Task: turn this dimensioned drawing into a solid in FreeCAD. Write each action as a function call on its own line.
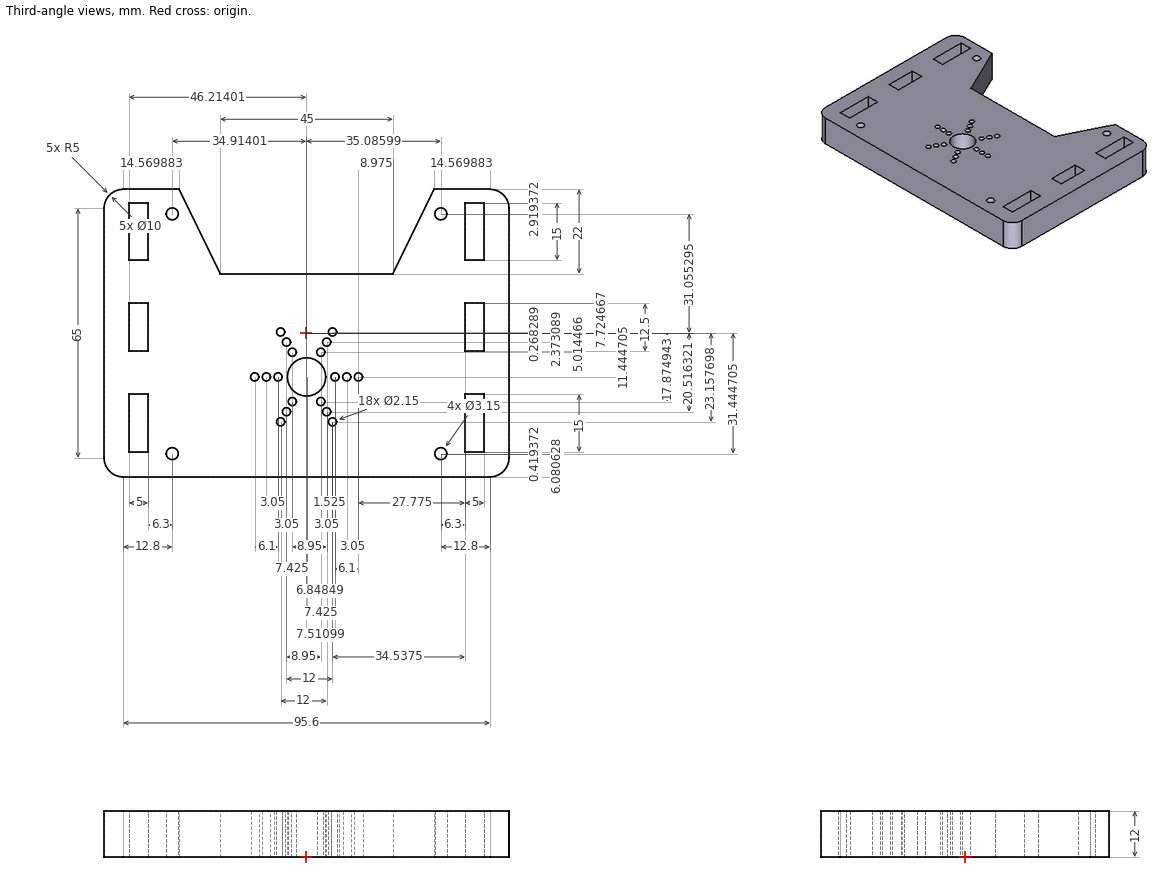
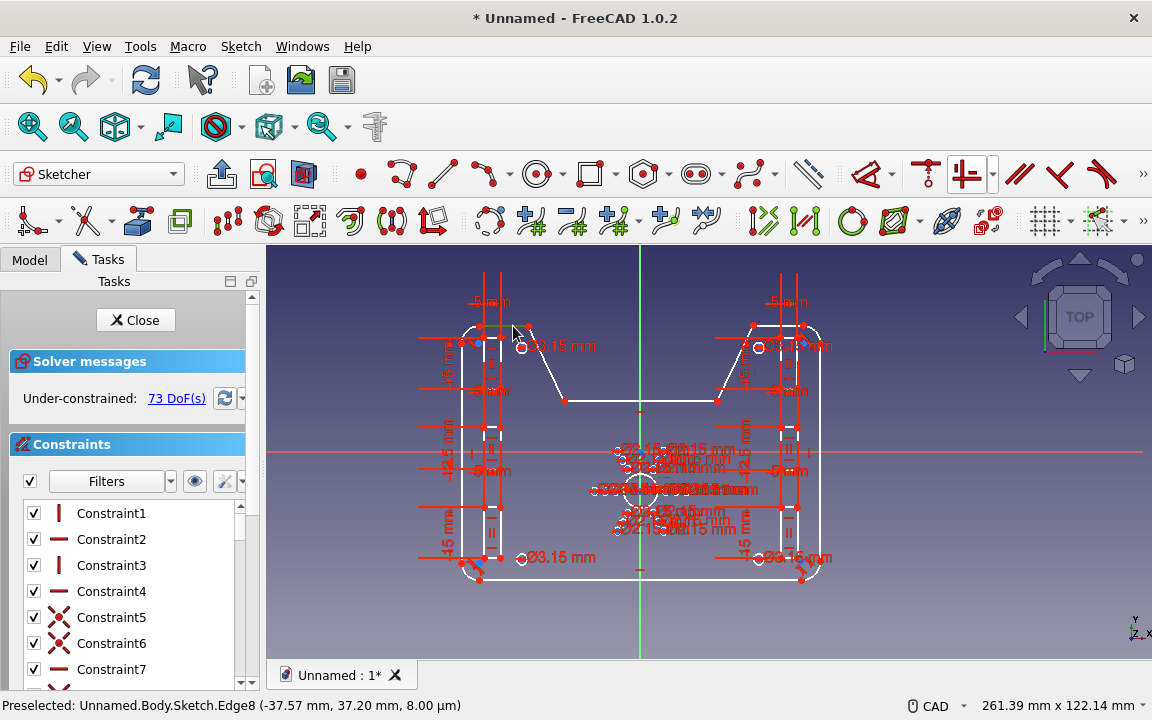
click(467, 331)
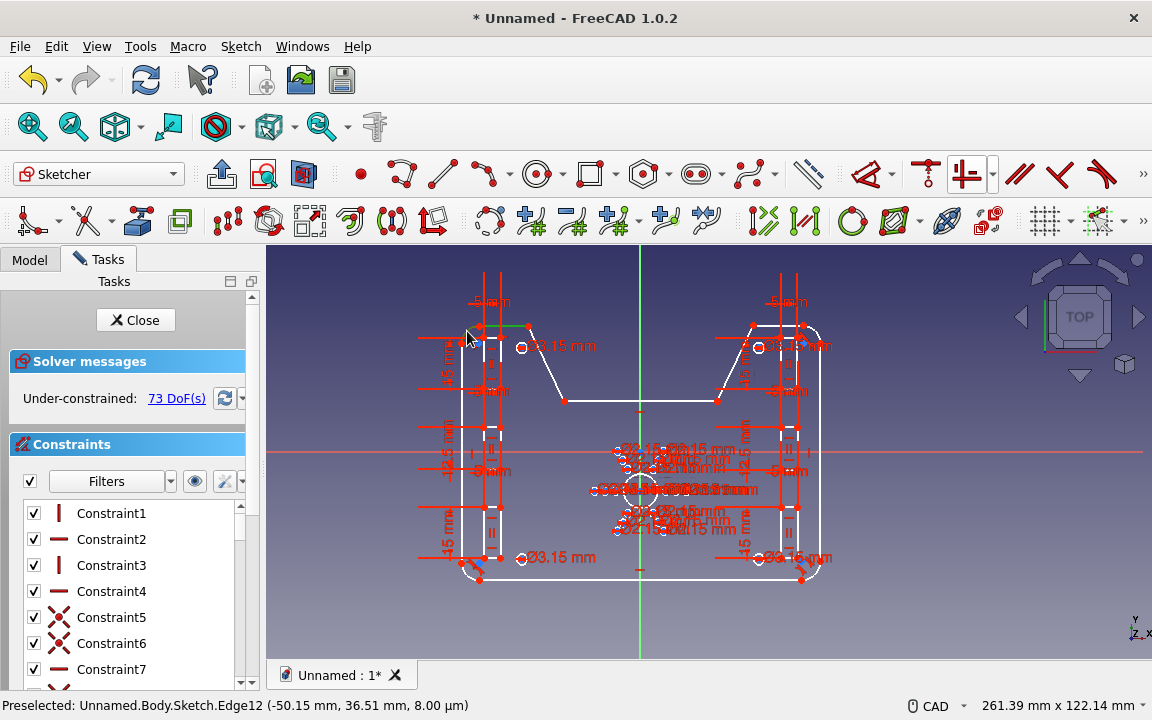
click(1102, 174)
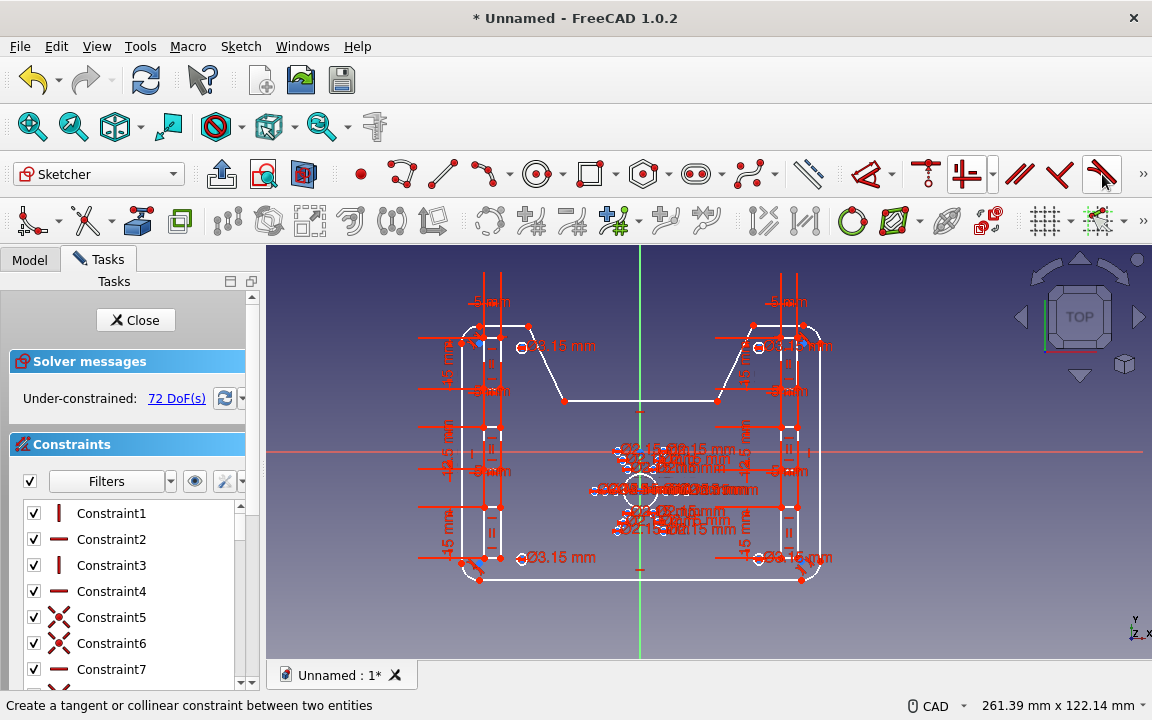
click(467, 575)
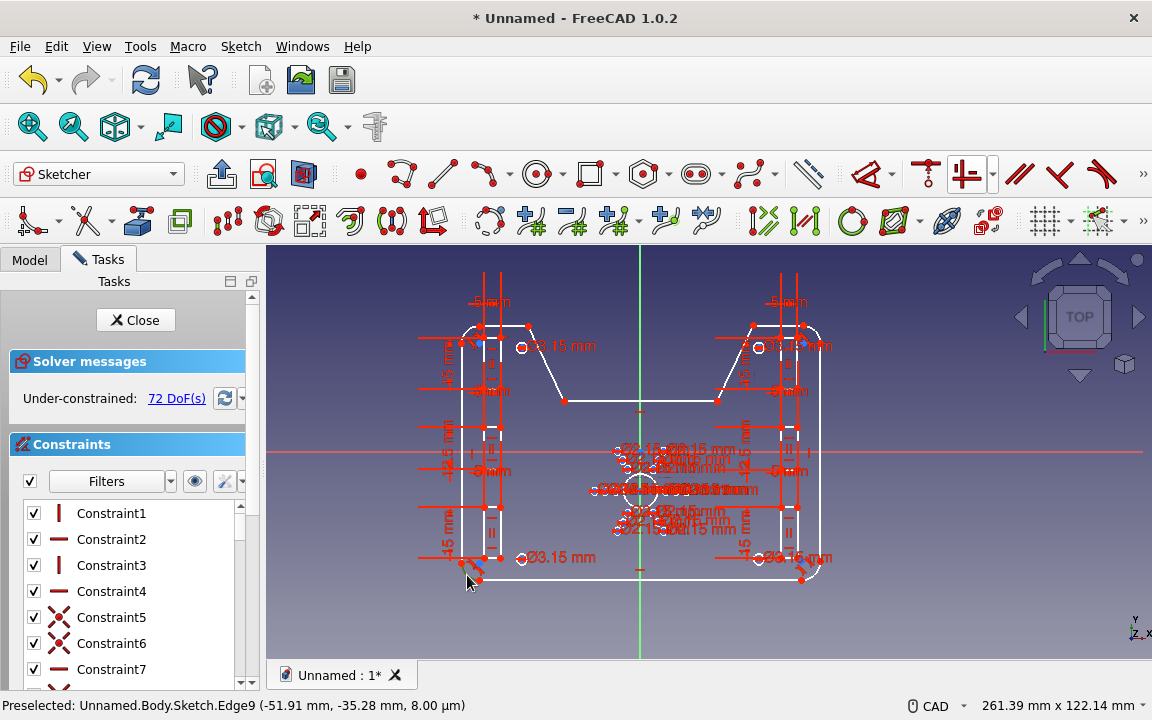
click(815, 575)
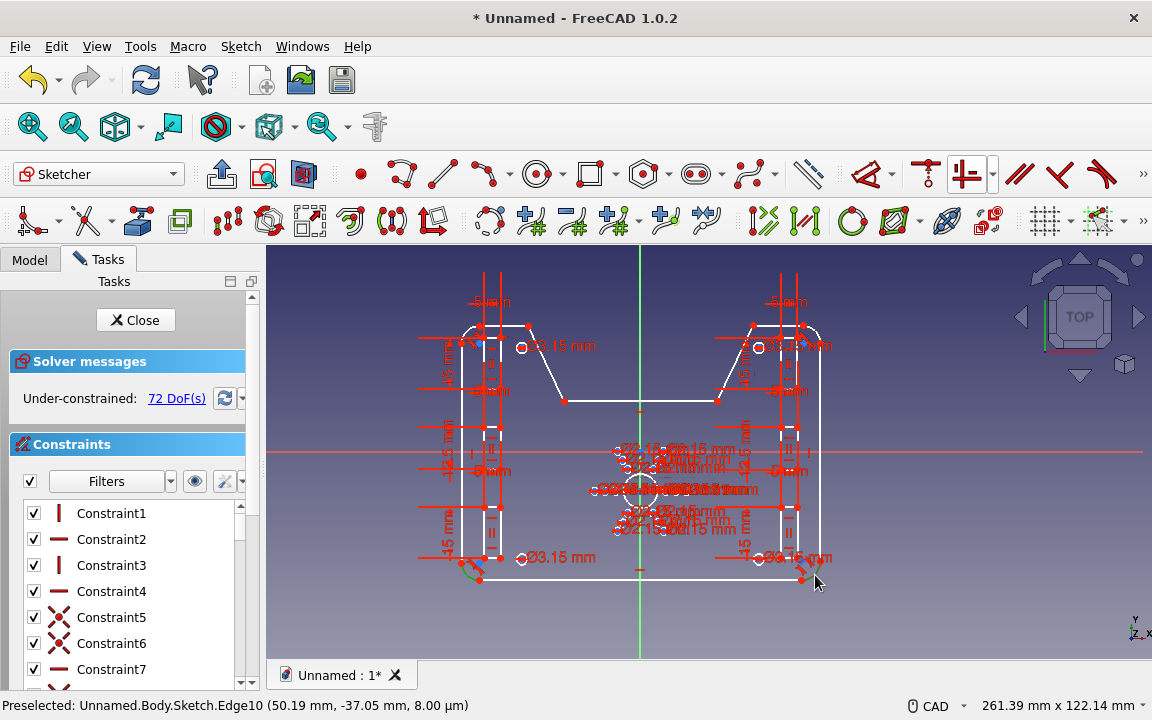
click(815, 331)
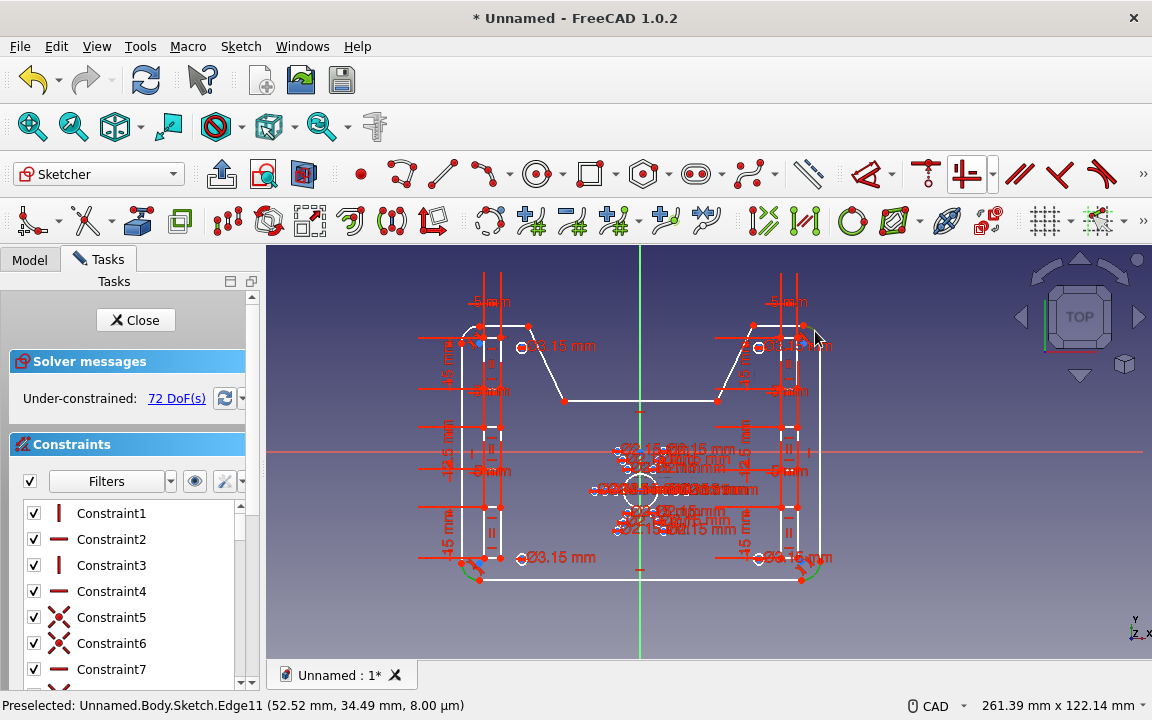
click(467, 331)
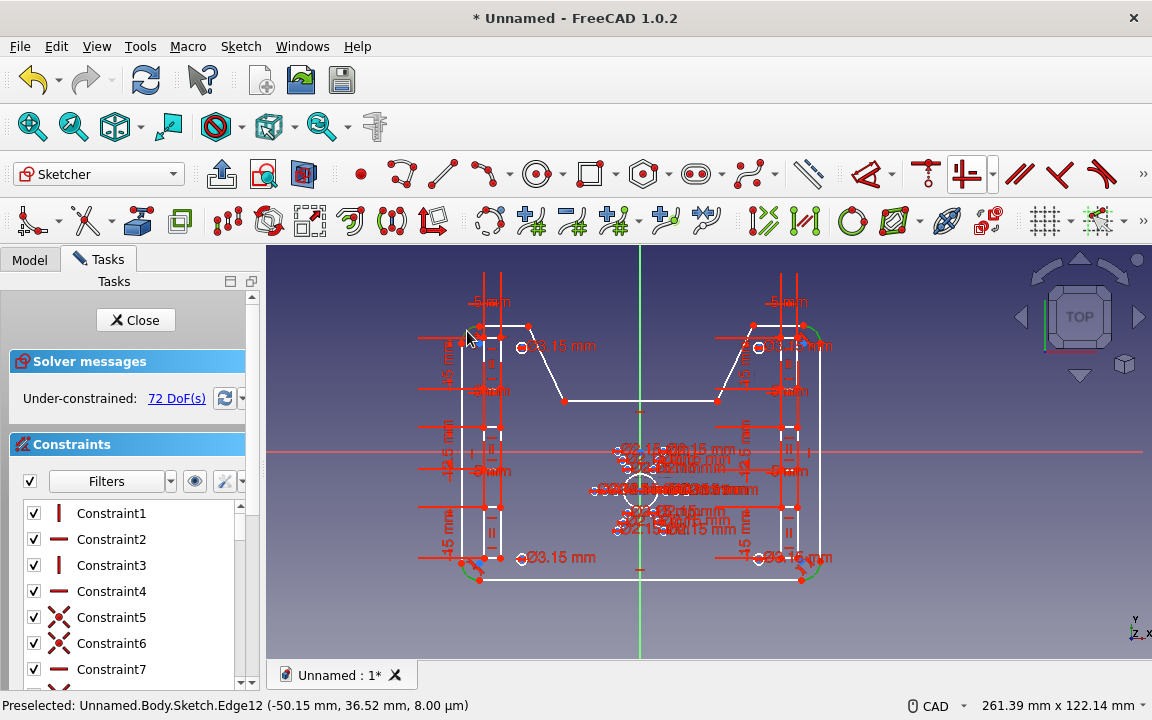
key(e)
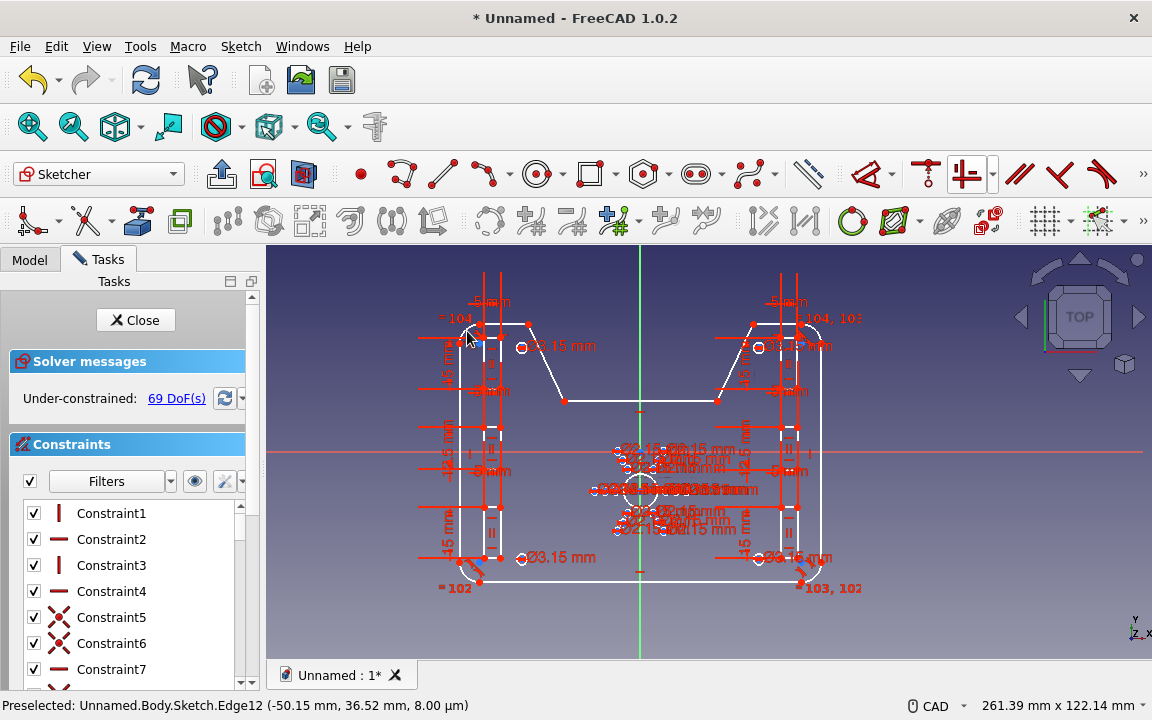
click(866, 174)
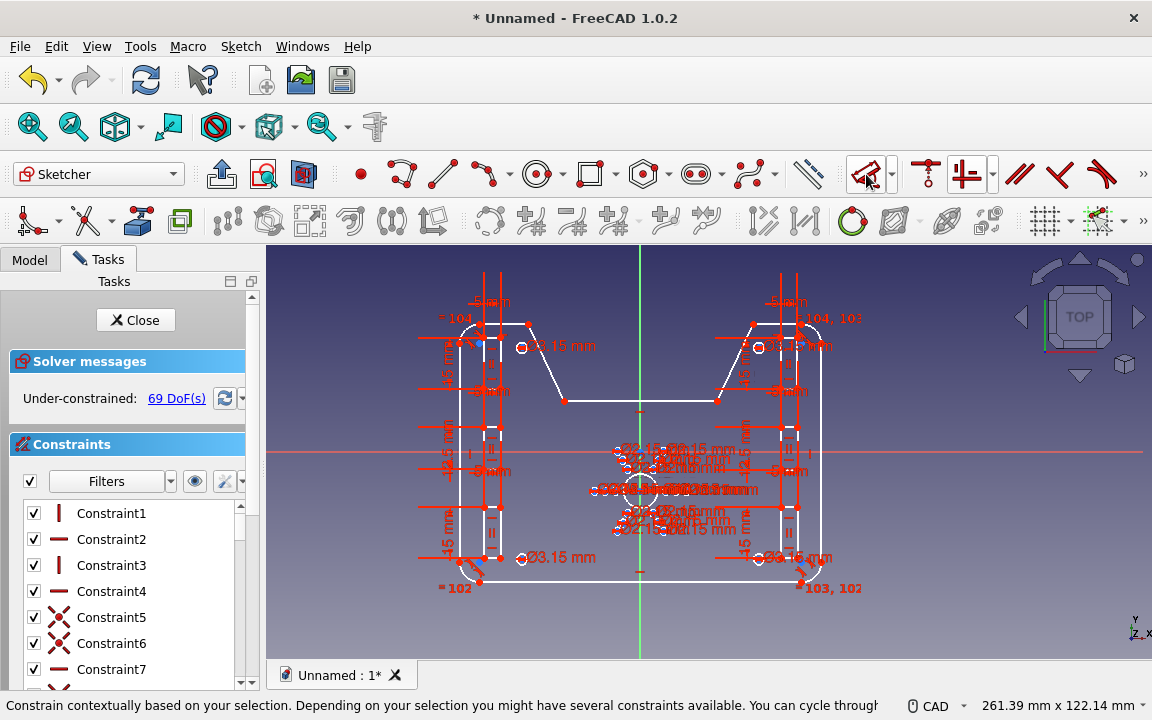
scroll(462, 572, up, 5)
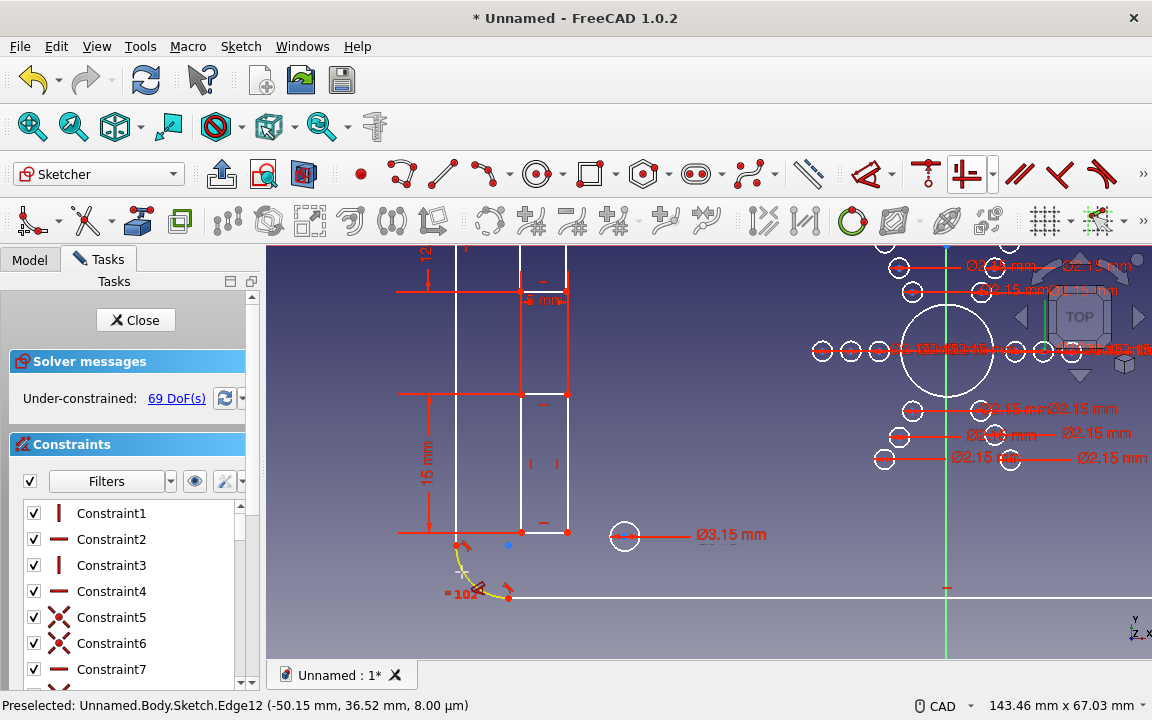
click(462, 569)
click(433, 583)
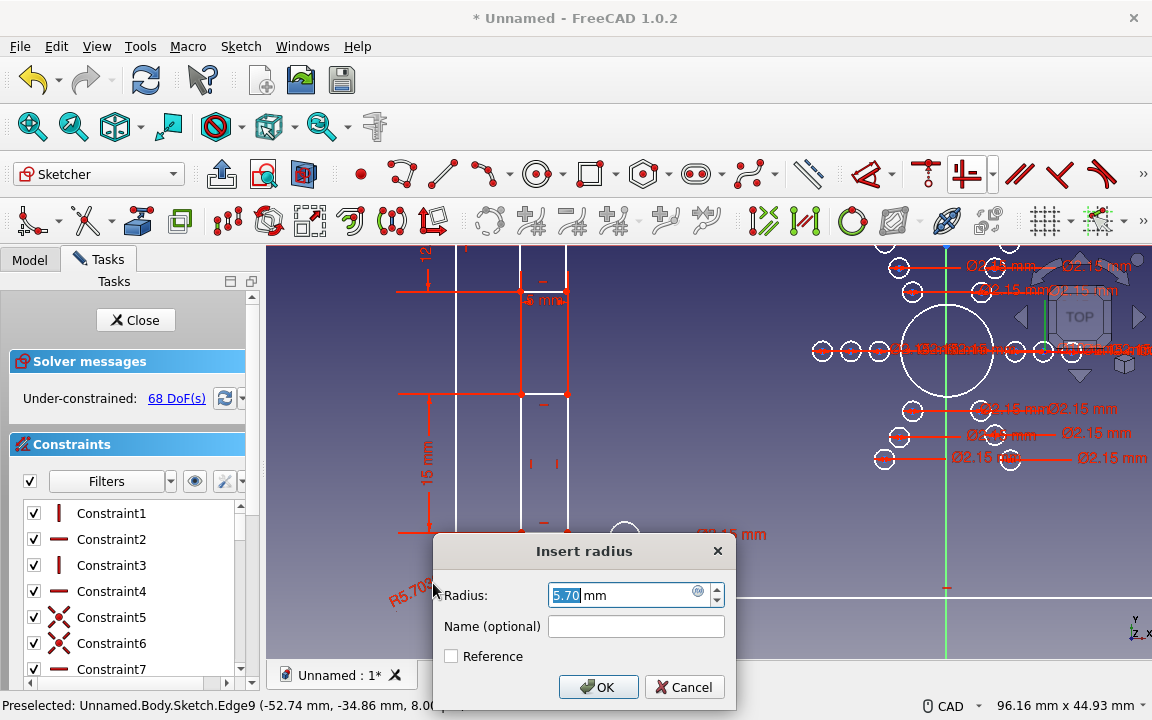
text(5)
key(Return)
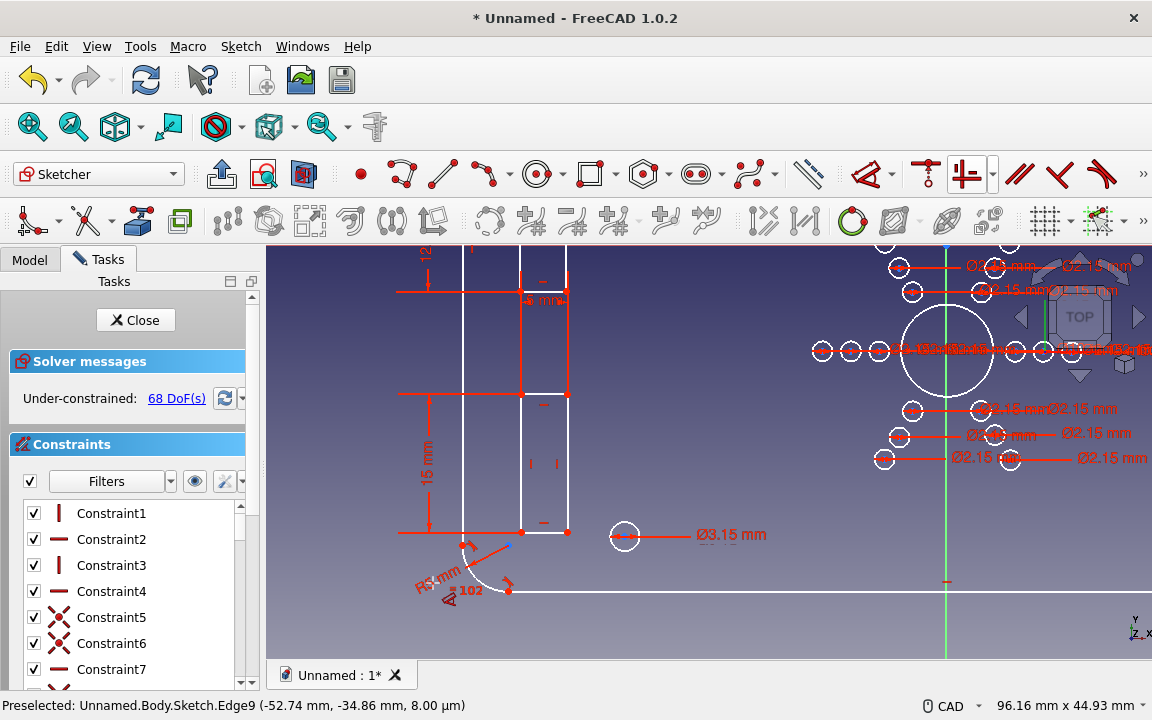
click(463, 367)
click(429, 409)